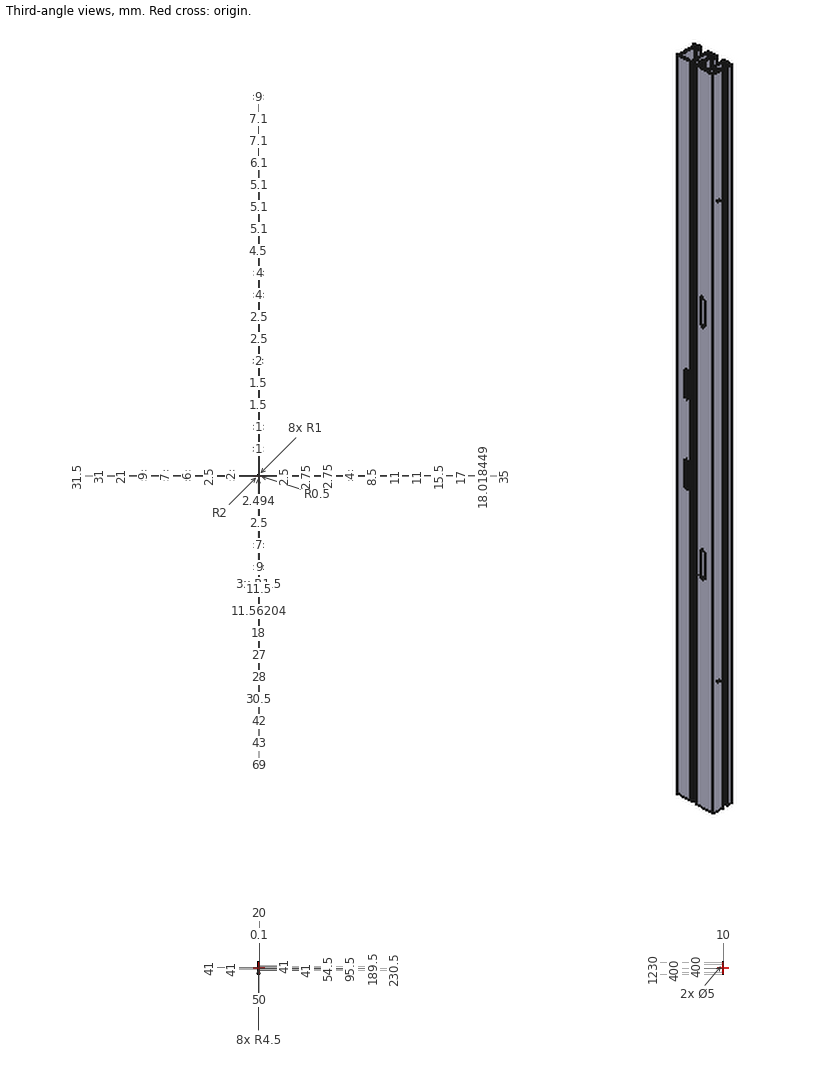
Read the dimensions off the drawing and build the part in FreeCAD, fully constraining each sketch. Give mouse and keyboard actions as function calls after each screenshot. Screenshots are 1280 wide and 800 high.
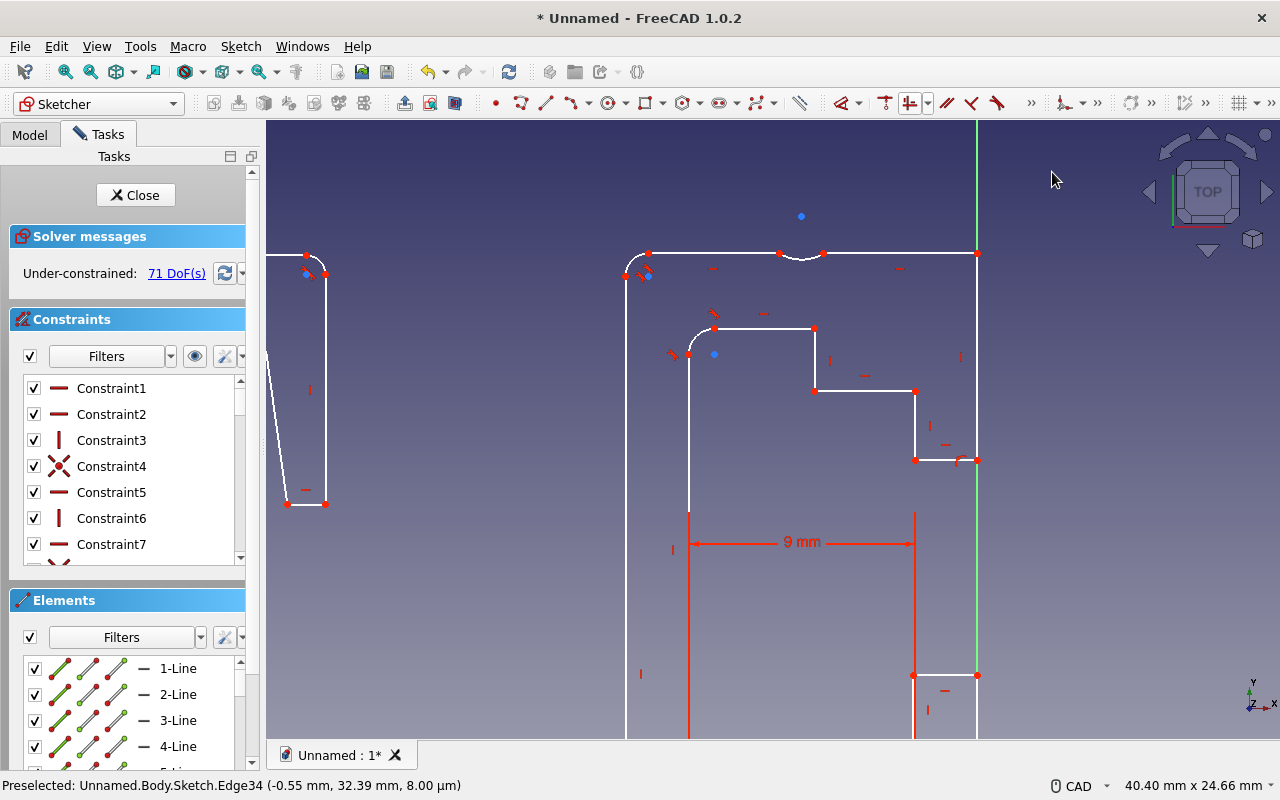
scroll(966, 317, down, 6)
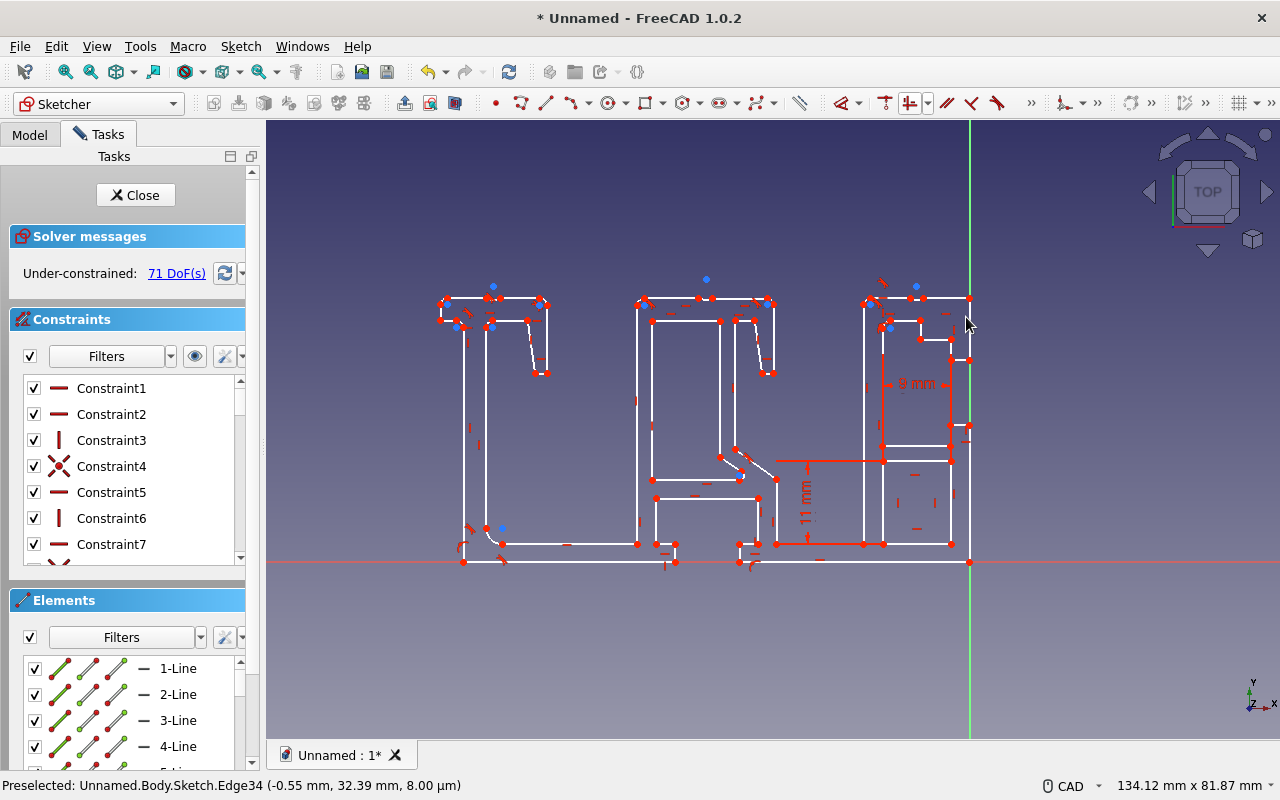
scroll(641, 299, up, 7)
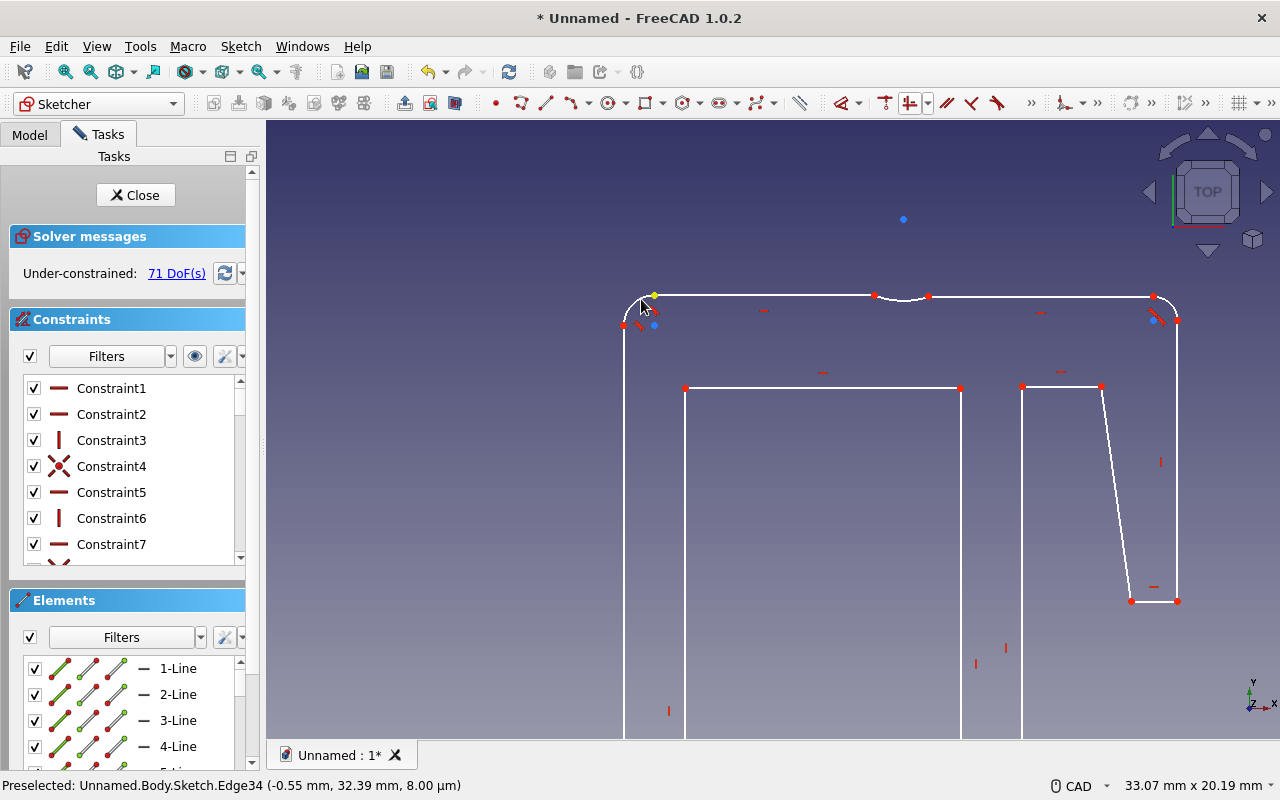
click(640, 299)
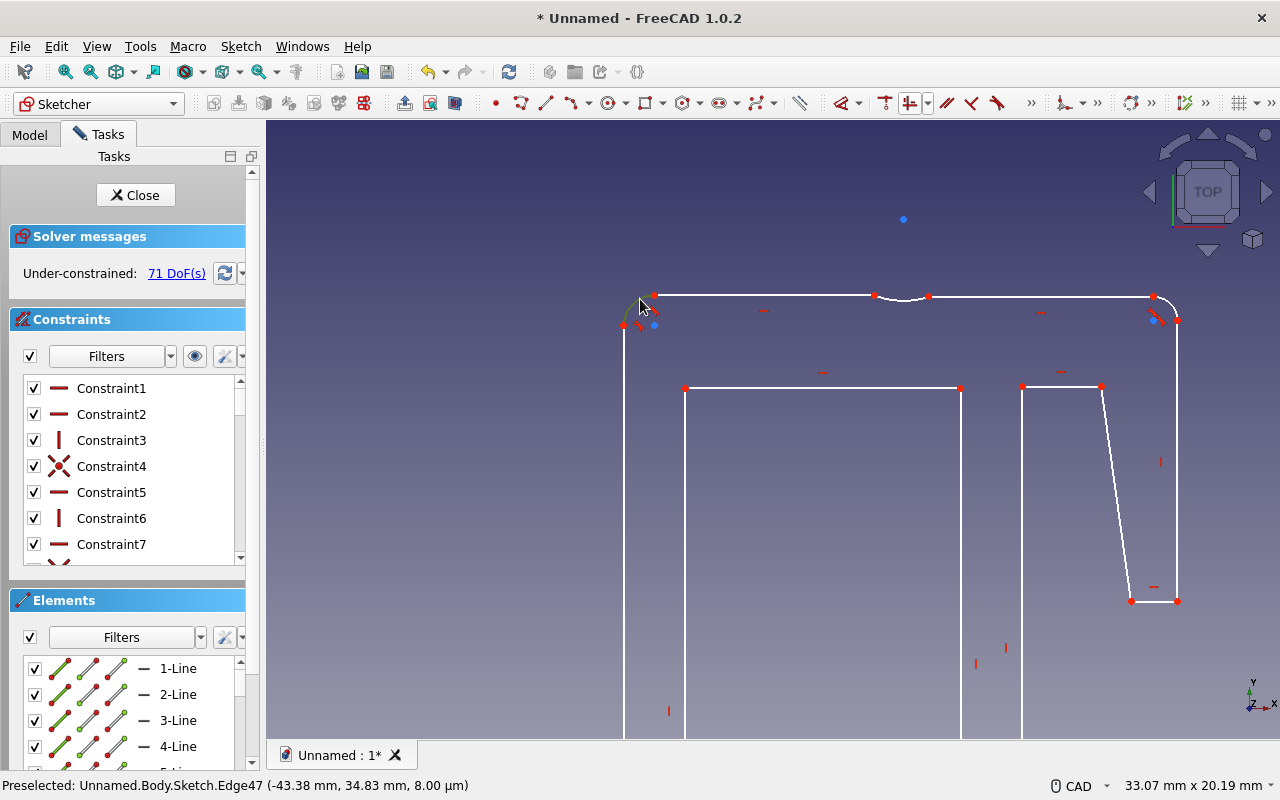
scroll(640, 299, down, 7)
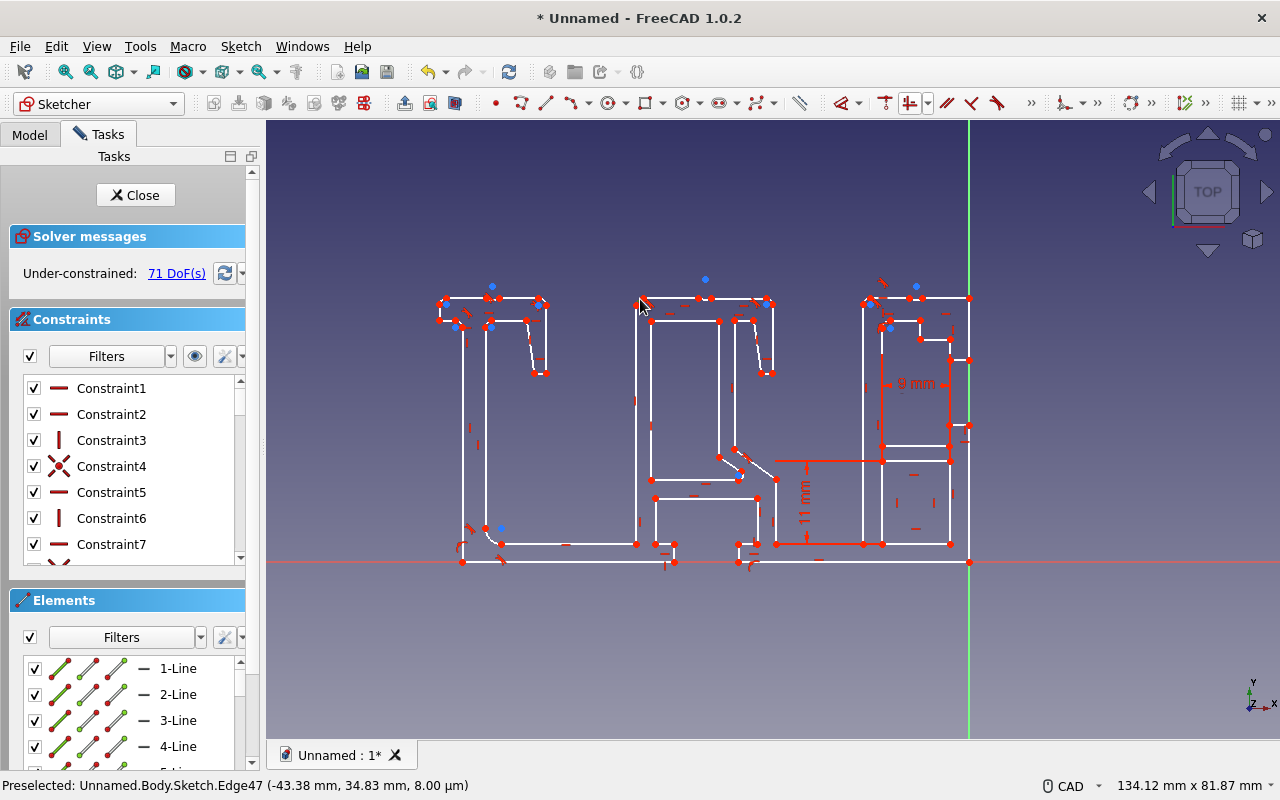
scroll(489, 322, up, 8)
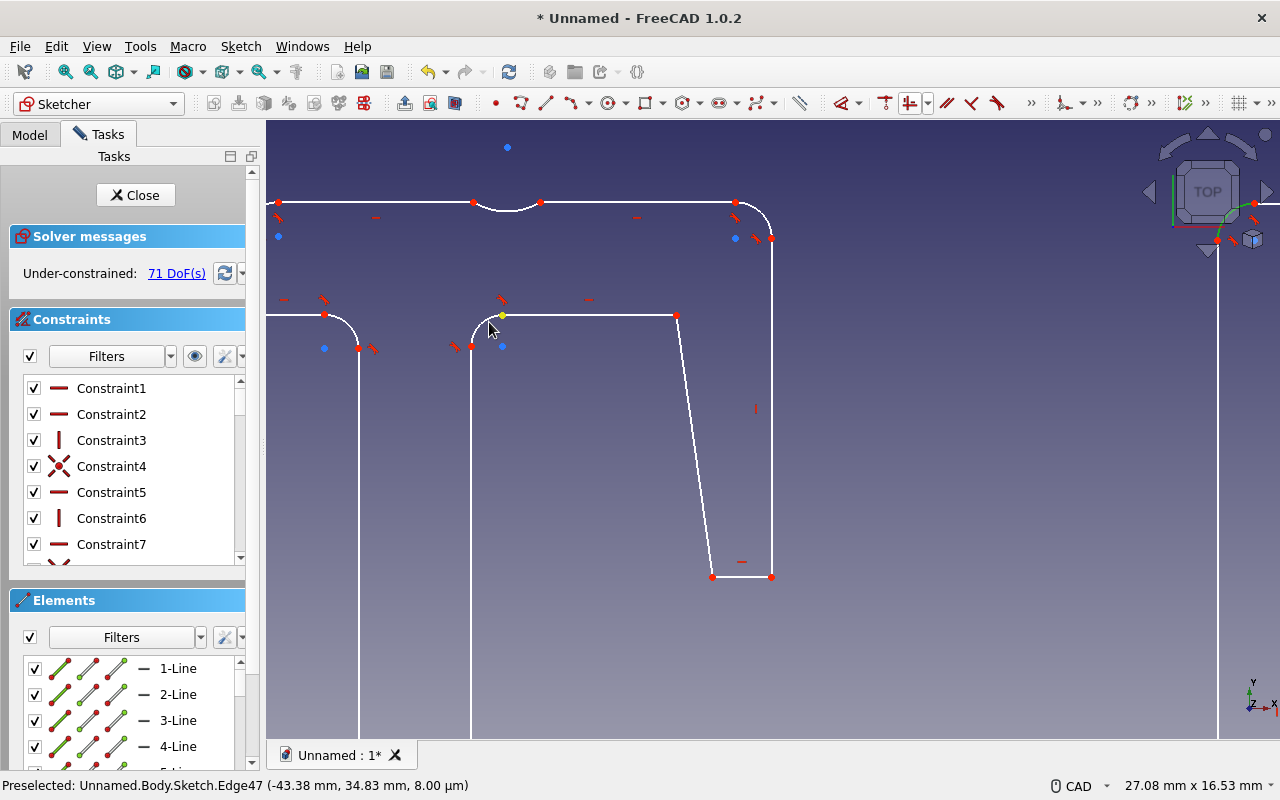
click(488, 319)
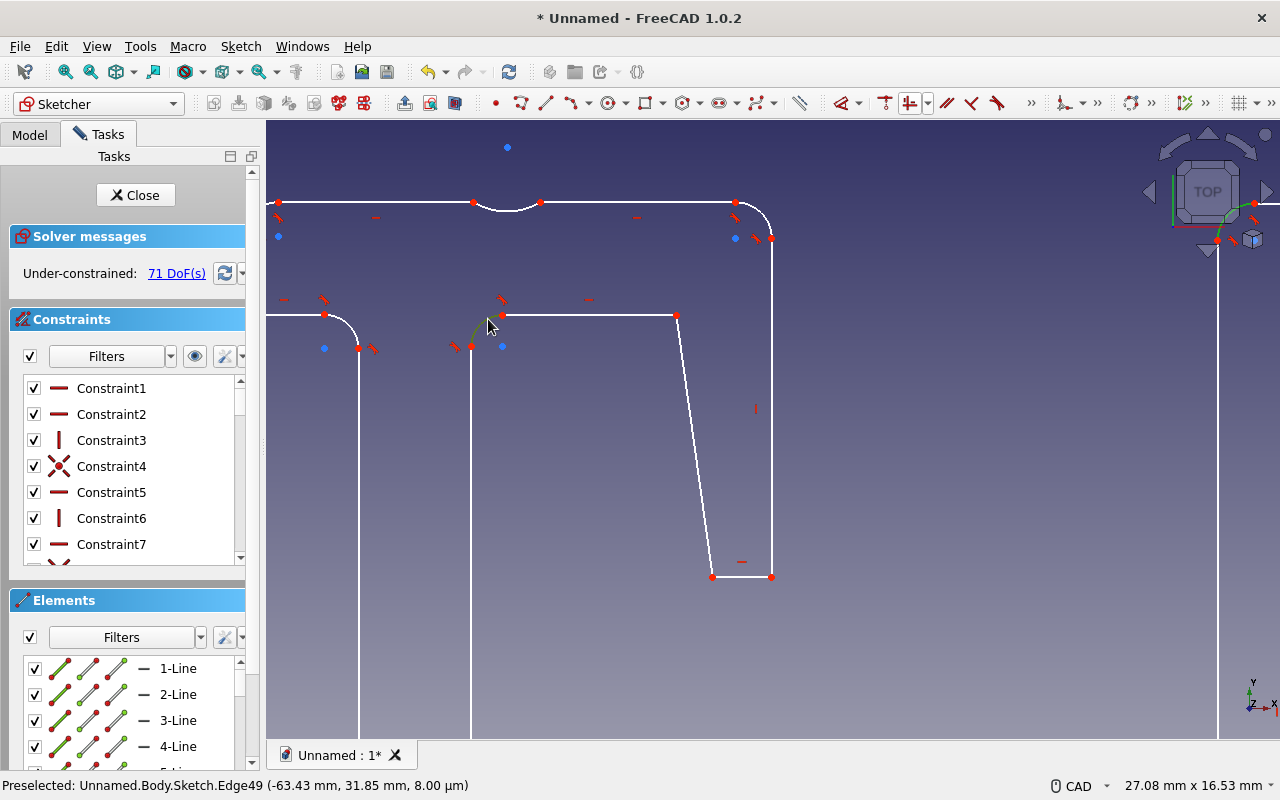
click(768, 222)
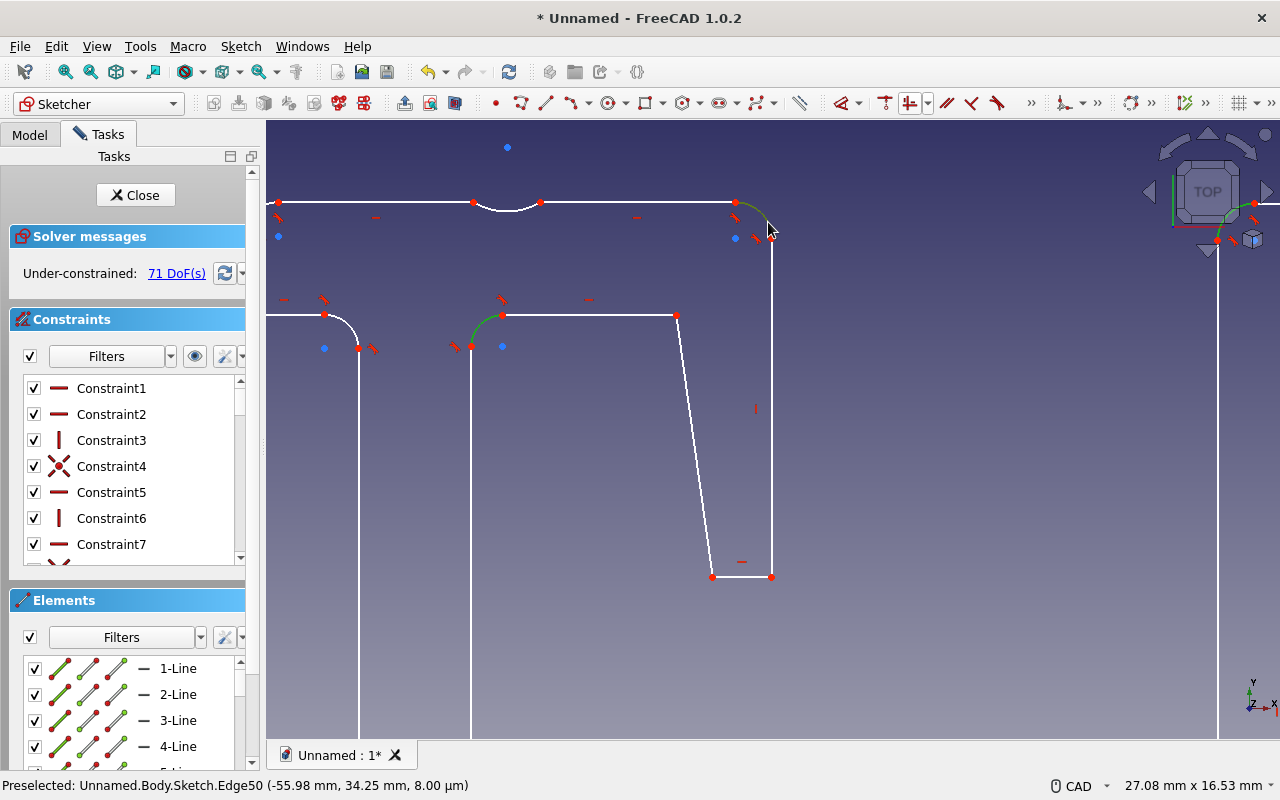
scroll(489, 322, down, 8)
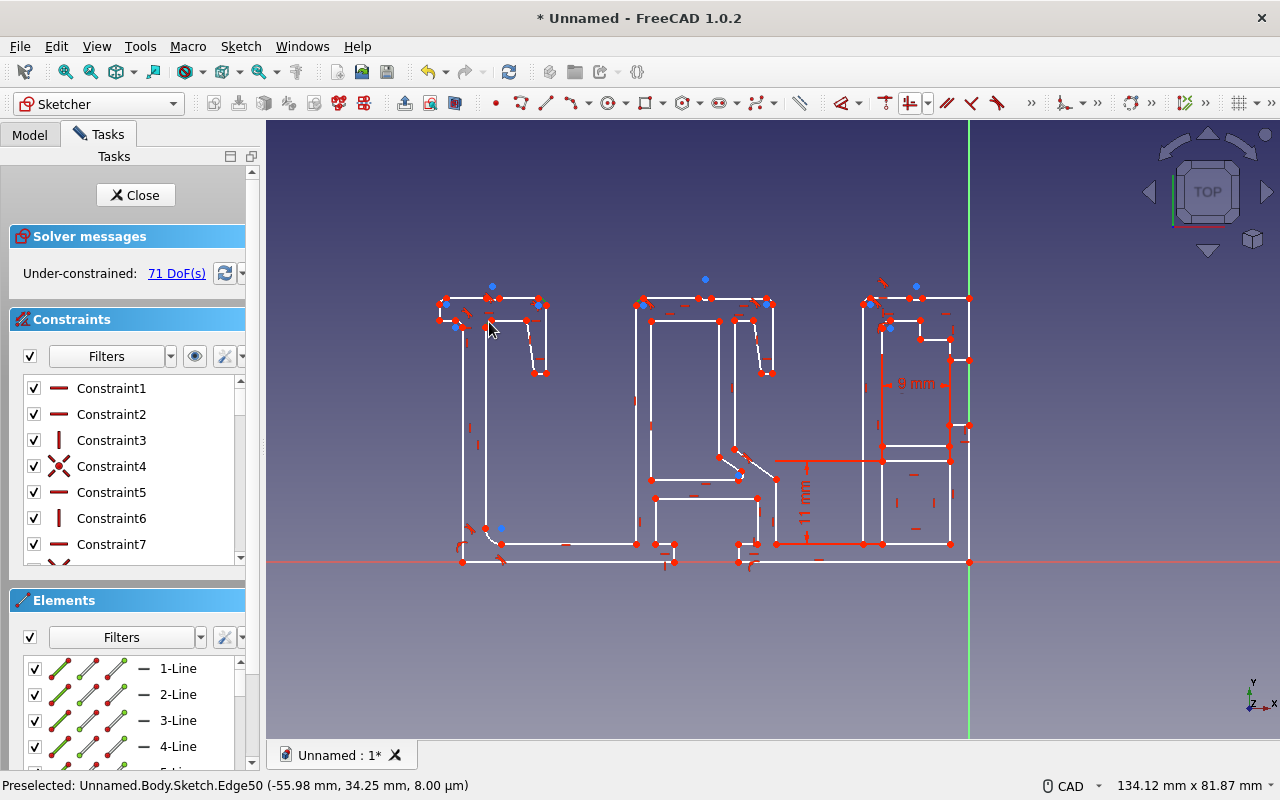
scroll(444, 299, up, 8)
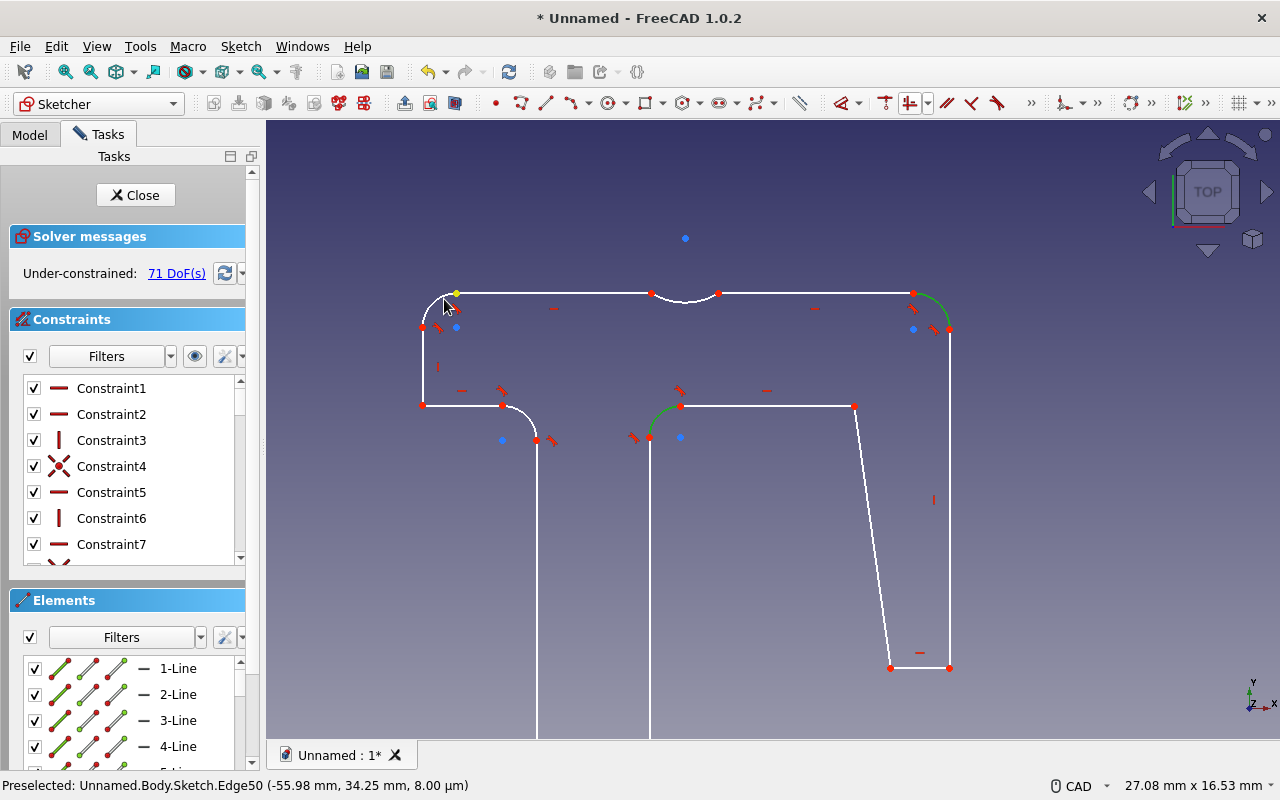
click(441, 297)